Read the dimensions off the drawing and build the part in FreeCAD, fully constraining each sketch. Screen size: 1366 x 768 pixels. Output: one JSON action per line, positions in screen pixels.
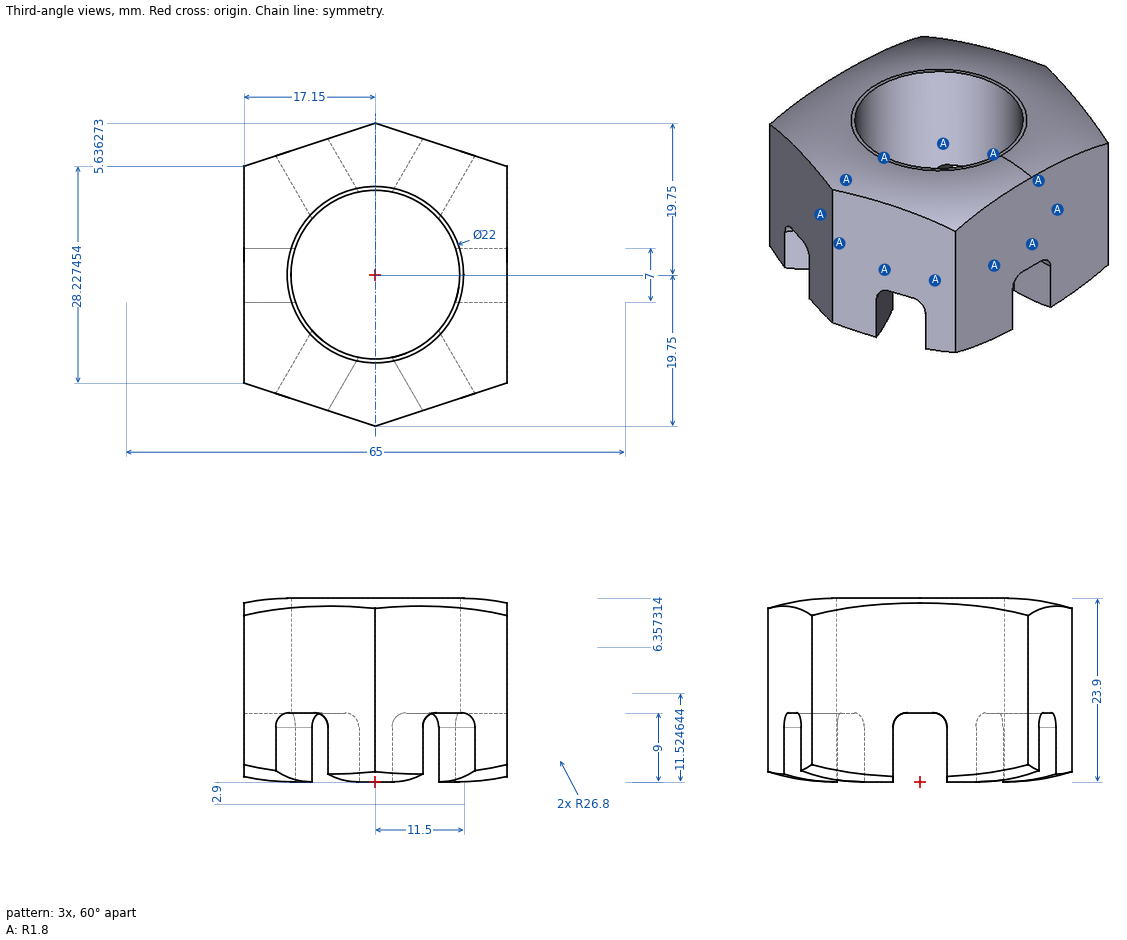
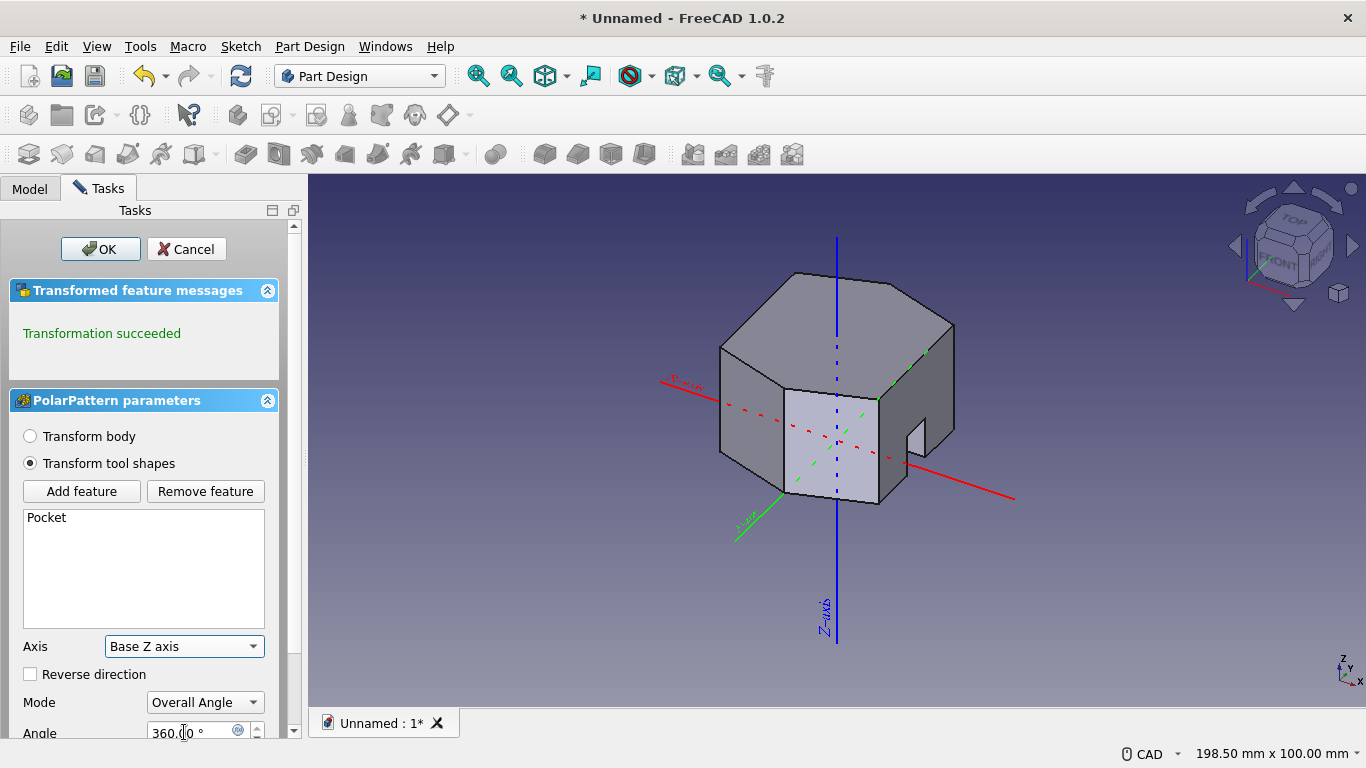
{"action": "left_click", "coordinate": [206, 702]}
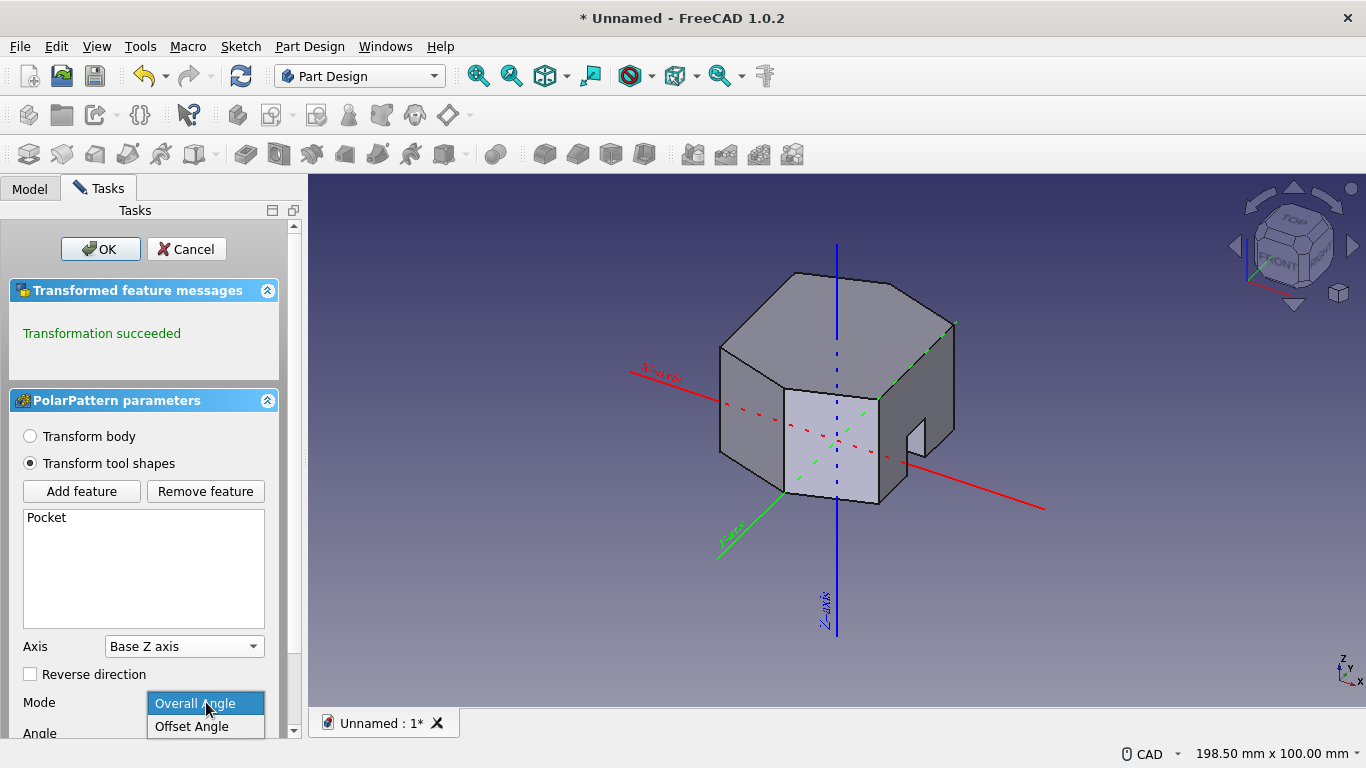
{"action": "left_click", "coordinate": [204, 726]}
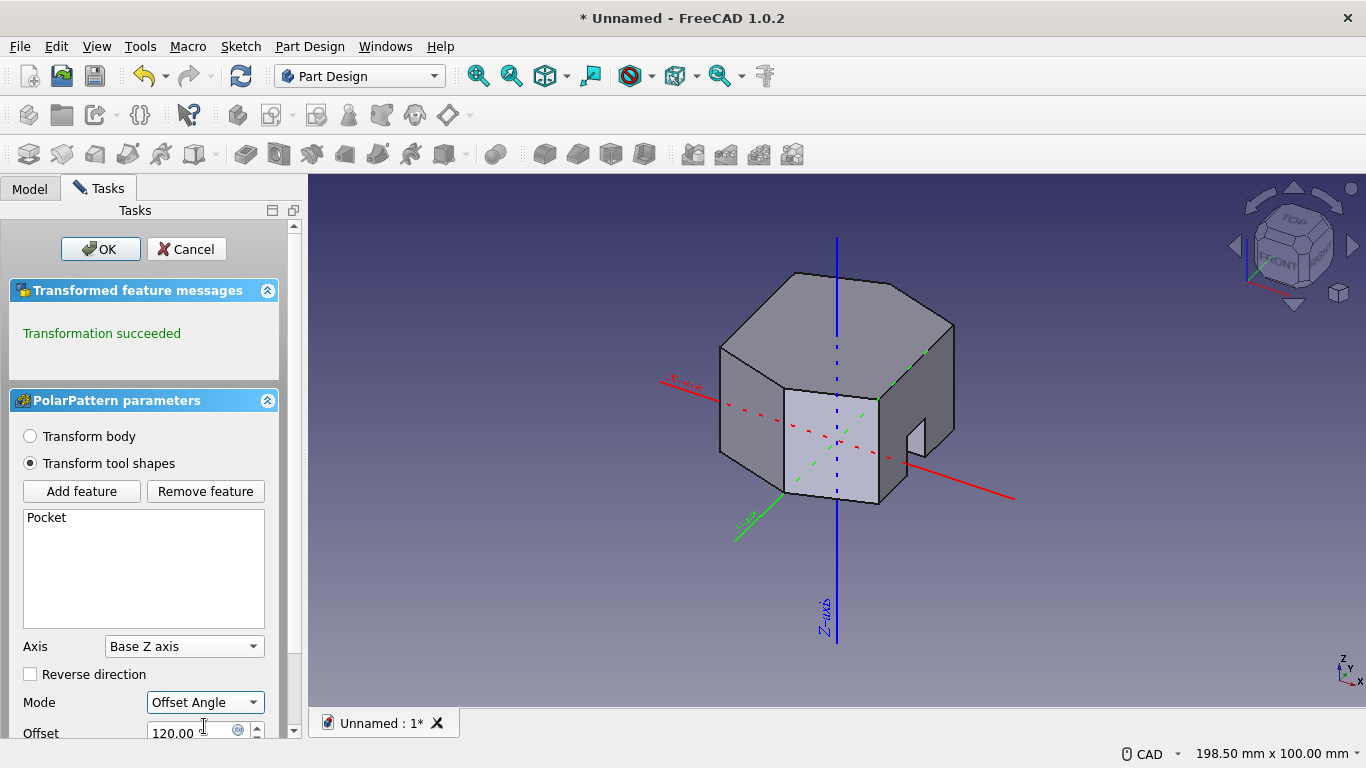
{"action": "scroll", "coordinate": [294, 479], "scroll_direction": "down", "scroll_amount": 2}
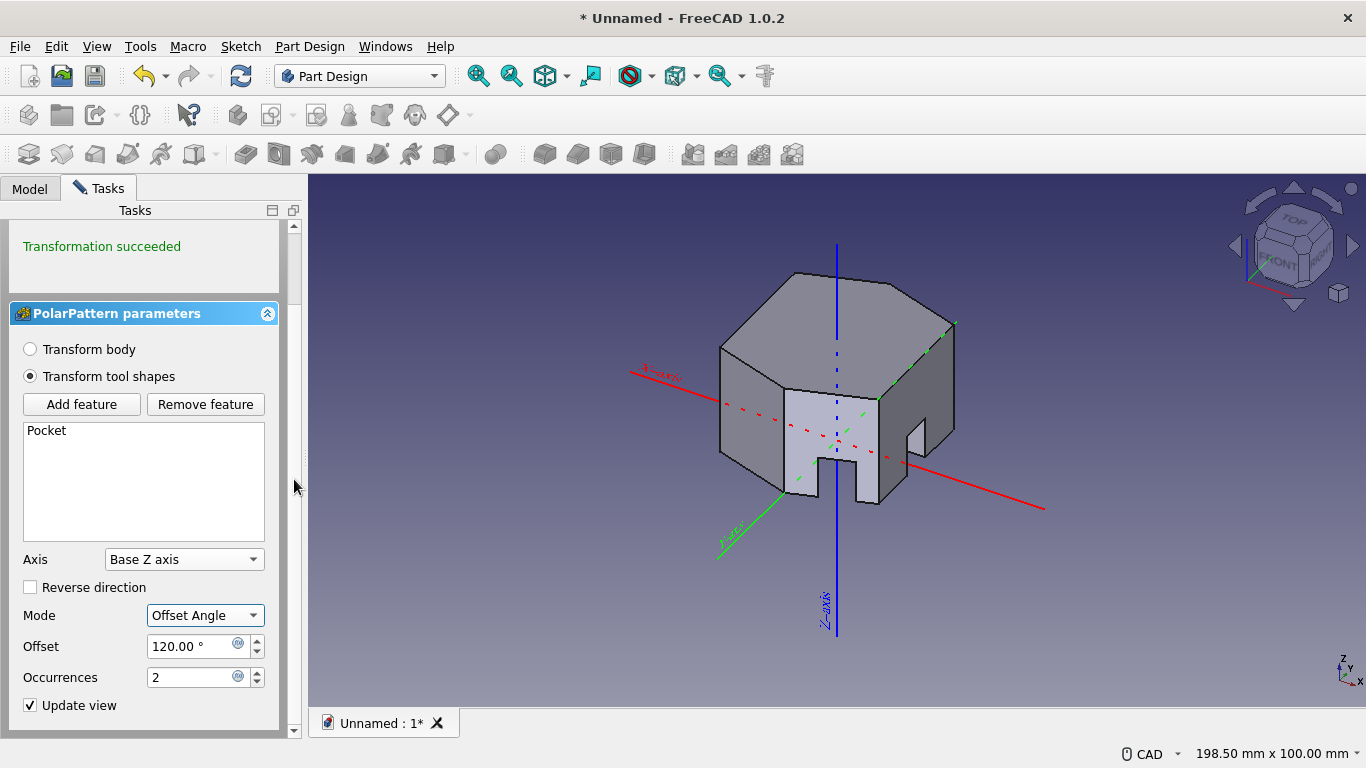
{"action": "triple_click", "coordinate": [199, 646]}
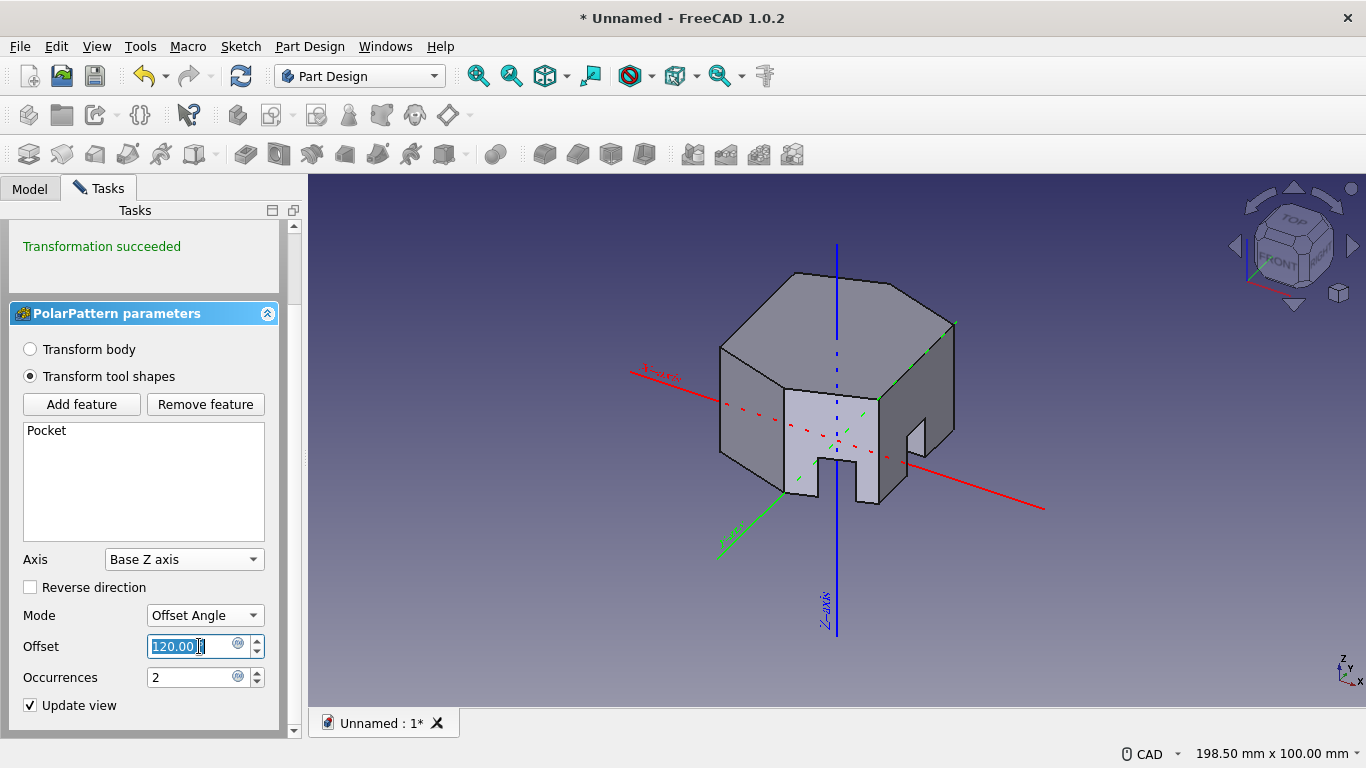
{"action": "type", "text": "60"}
{"action": "key", "text": "Tab"}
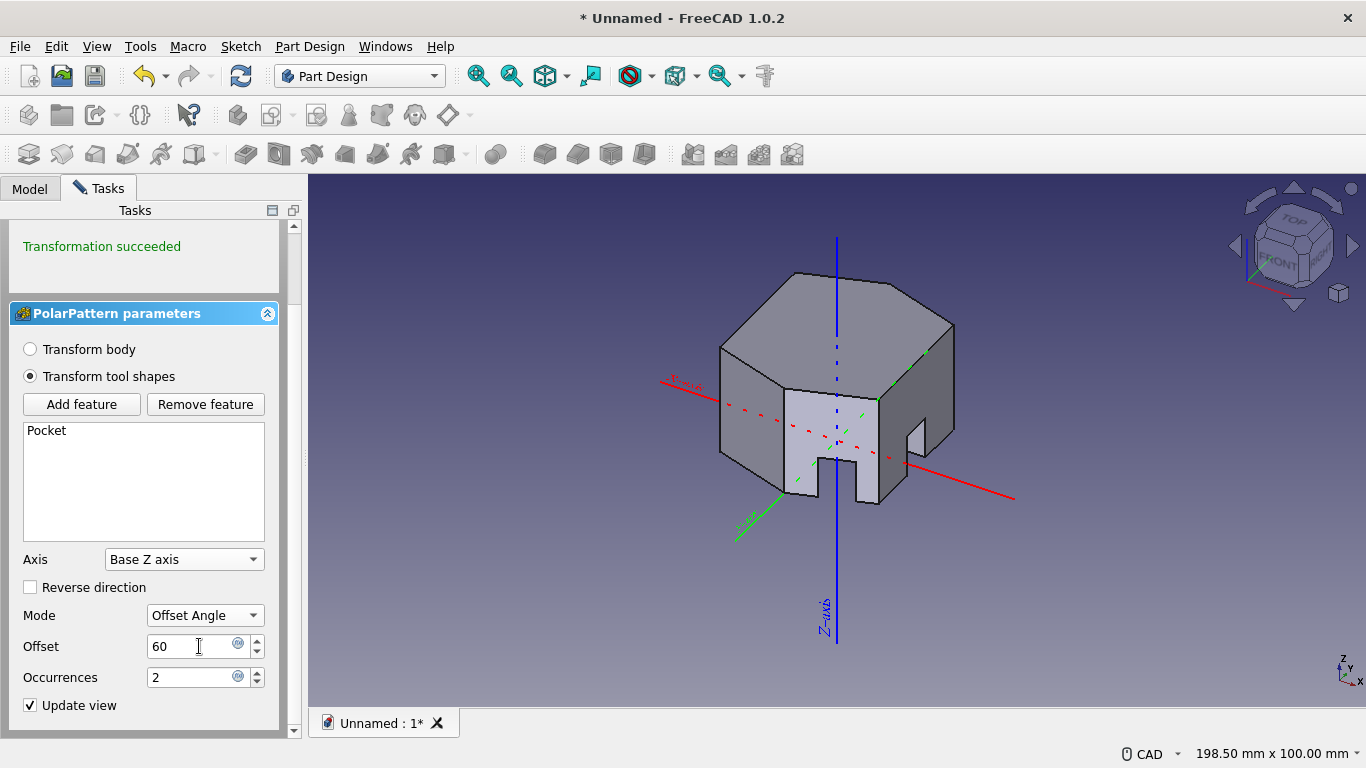
{"action": "triple_click", "coordinate": [199, 678]}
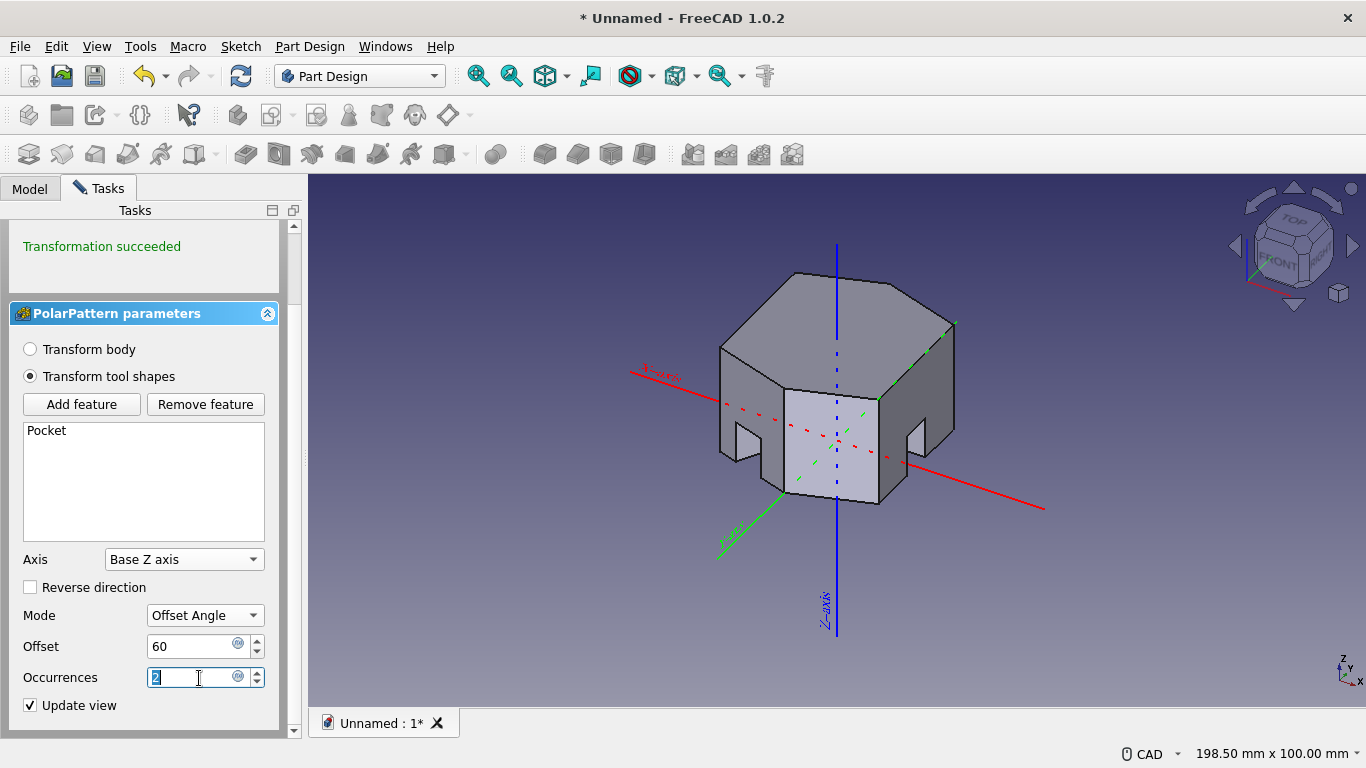
{"action": "type", "text": "3"}
{"action": "key", "text": "Tab"}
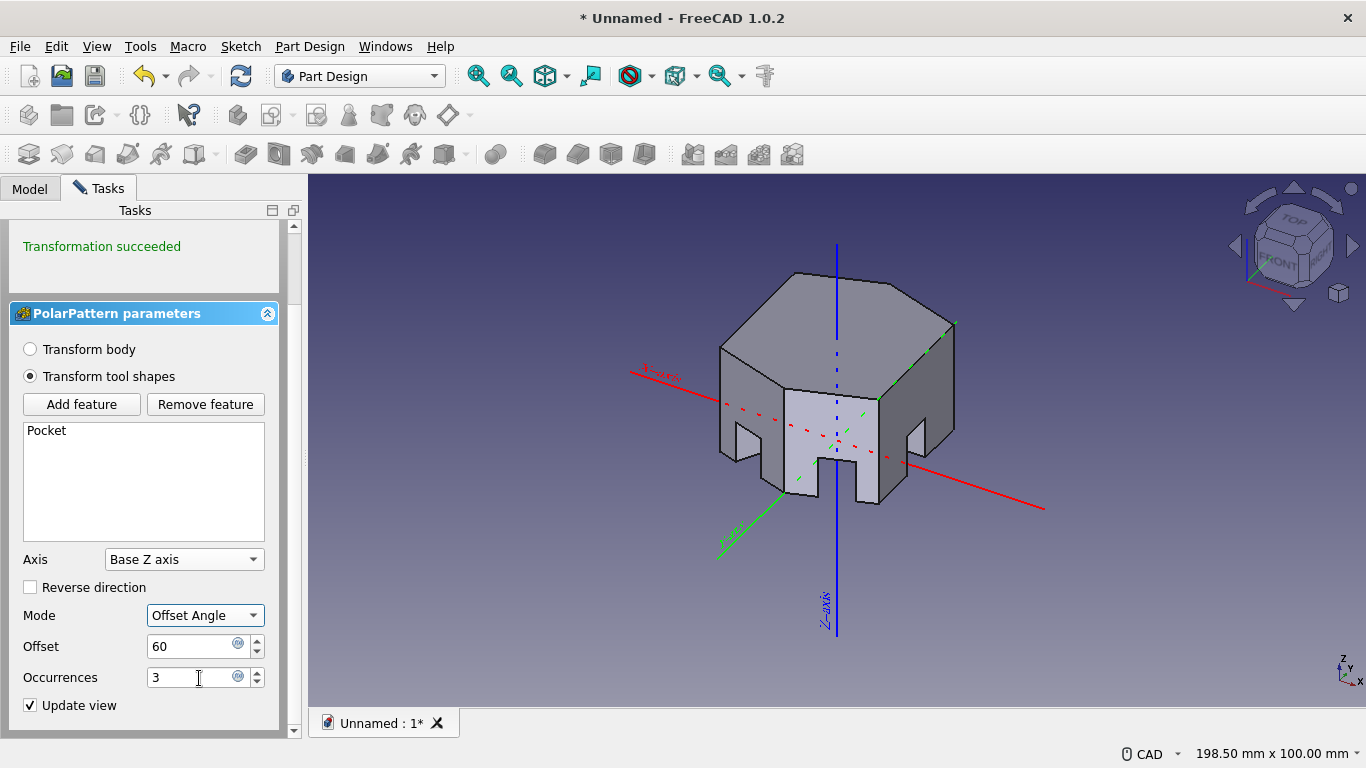
{"action": "scroll", "coordinate": [294, 479], "scroll_direction": "up", "scroll_amount": 3}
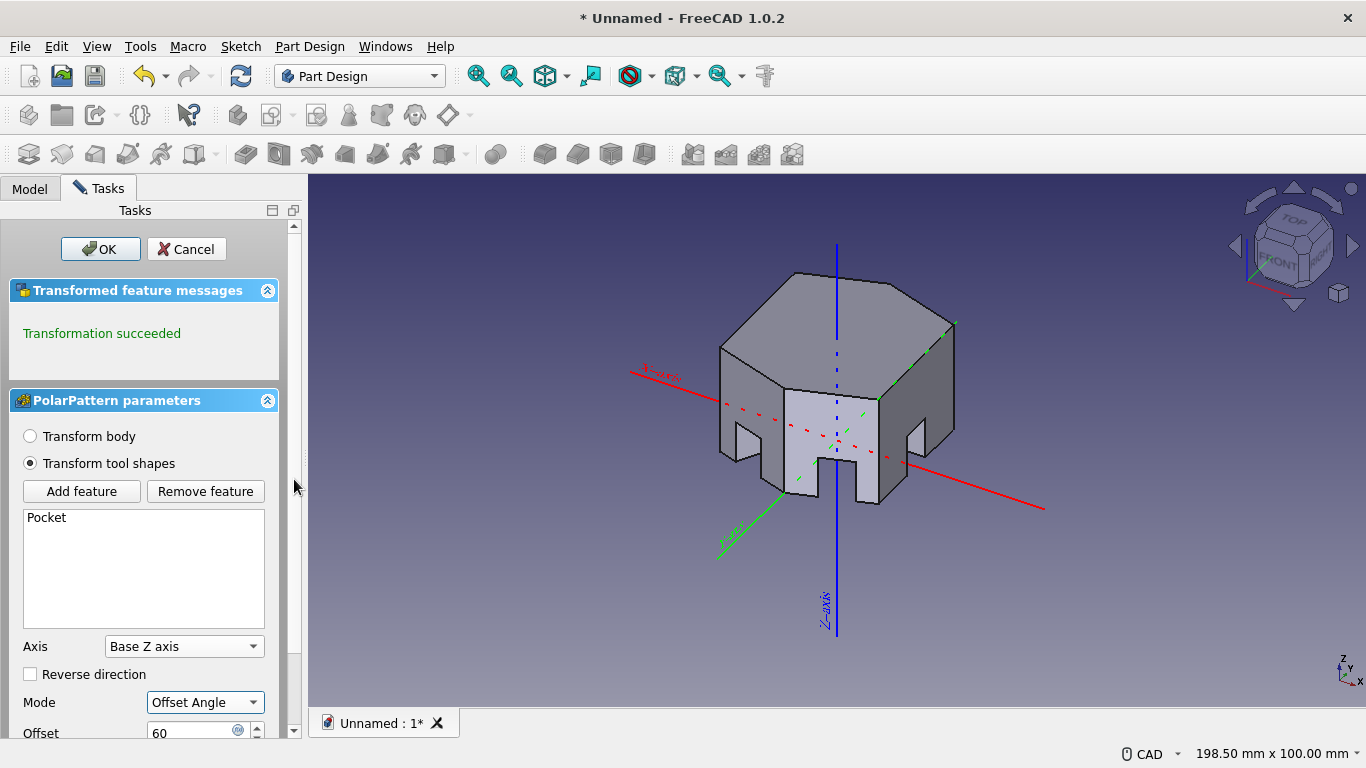
{"action": "left_click", "coordinate": [101, 249]}